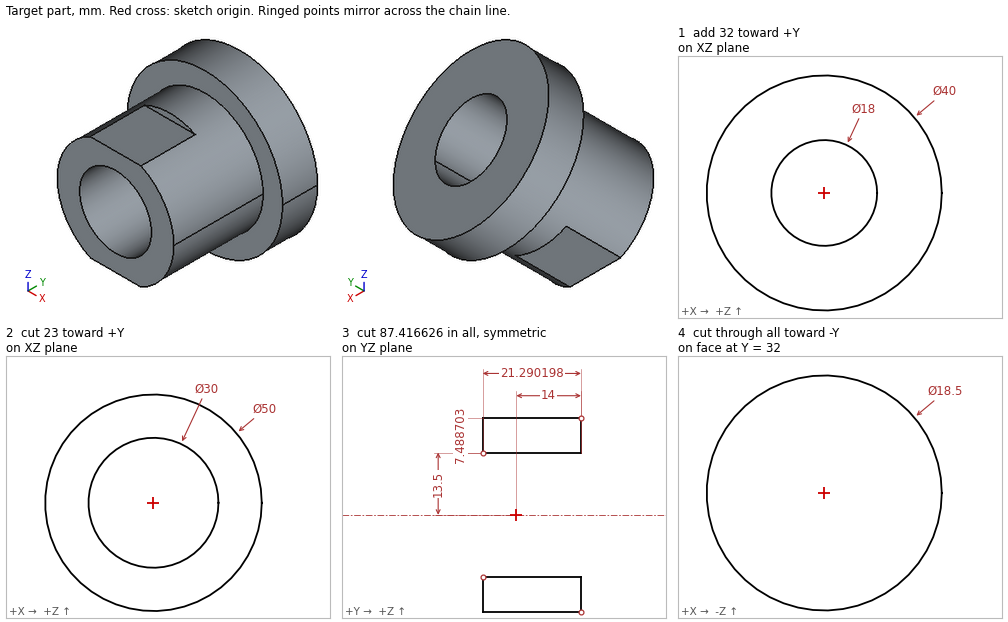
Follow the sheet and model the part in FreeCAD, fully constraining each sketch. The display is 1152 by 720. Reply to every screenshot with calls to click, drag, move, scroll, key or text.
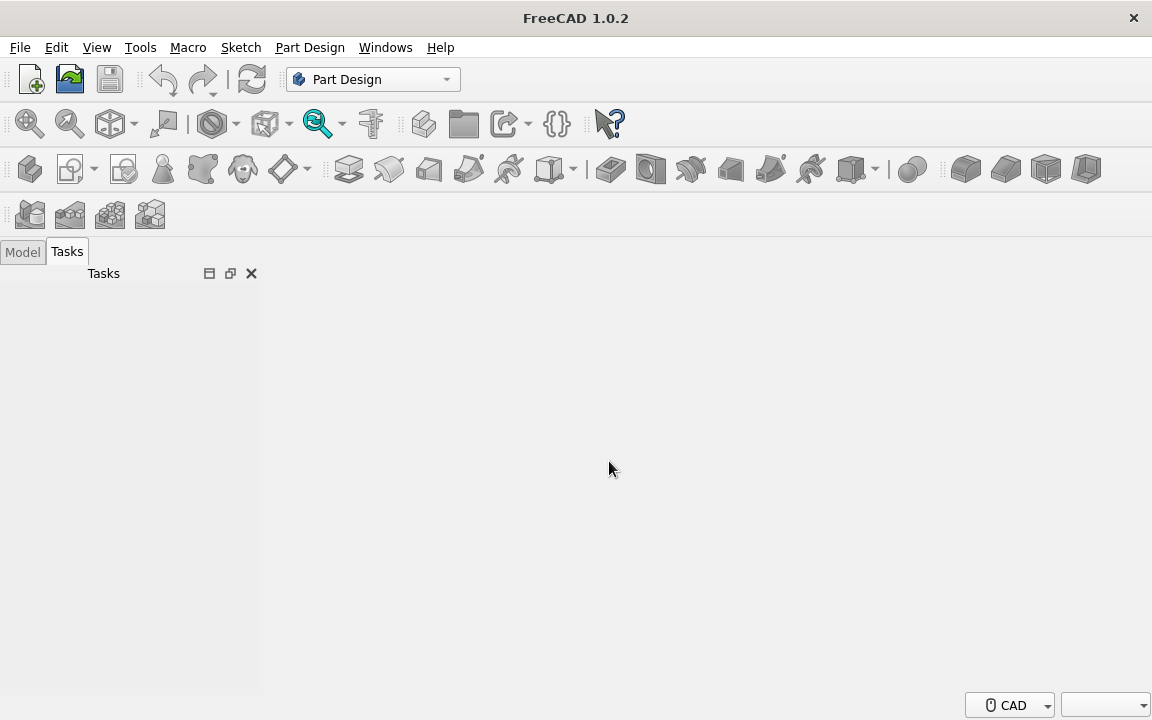
key(ctrl+n)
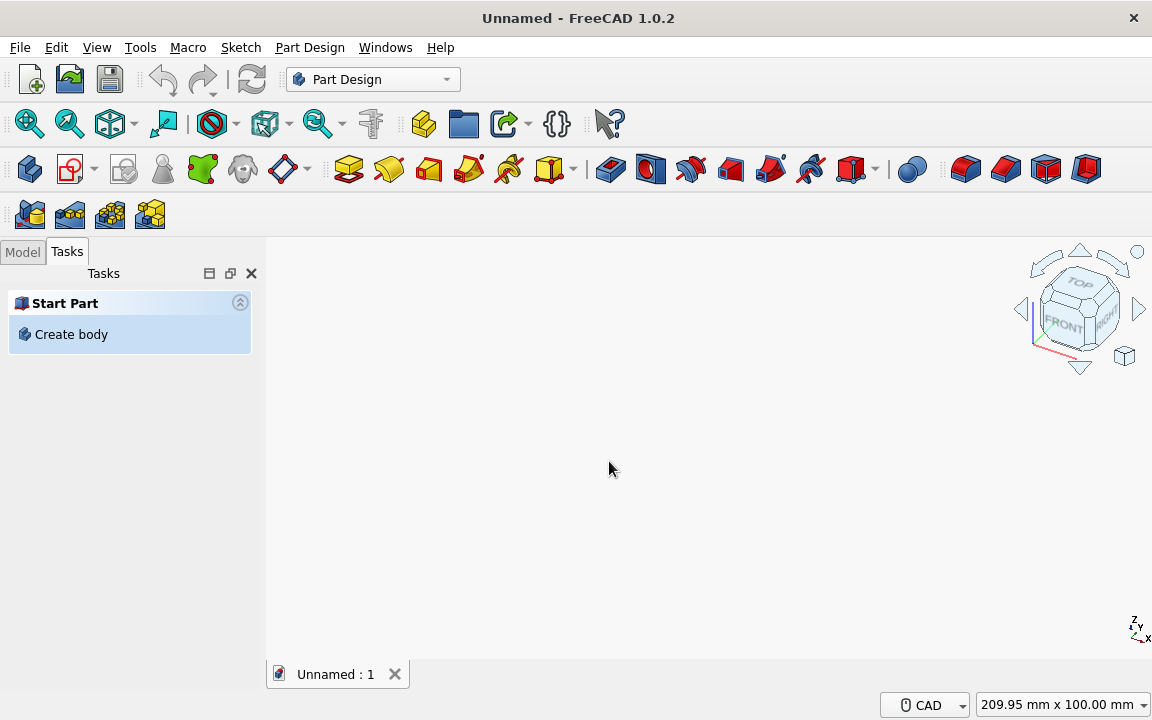
click(70, 170)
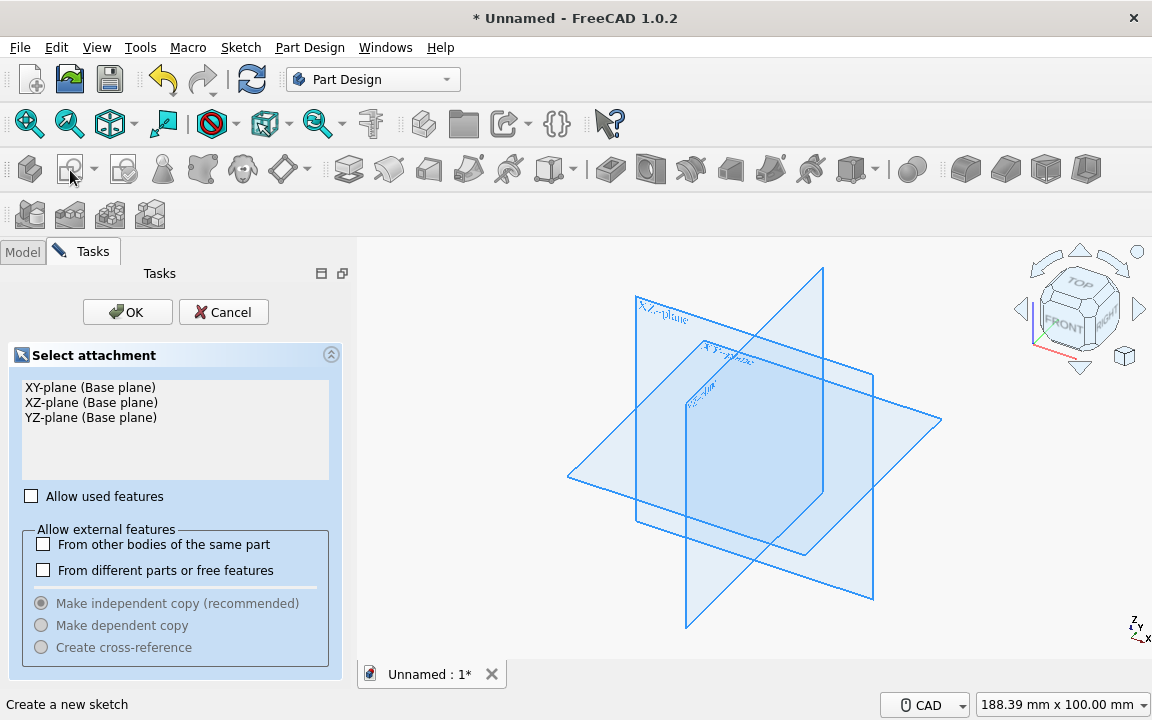
click(82, 402)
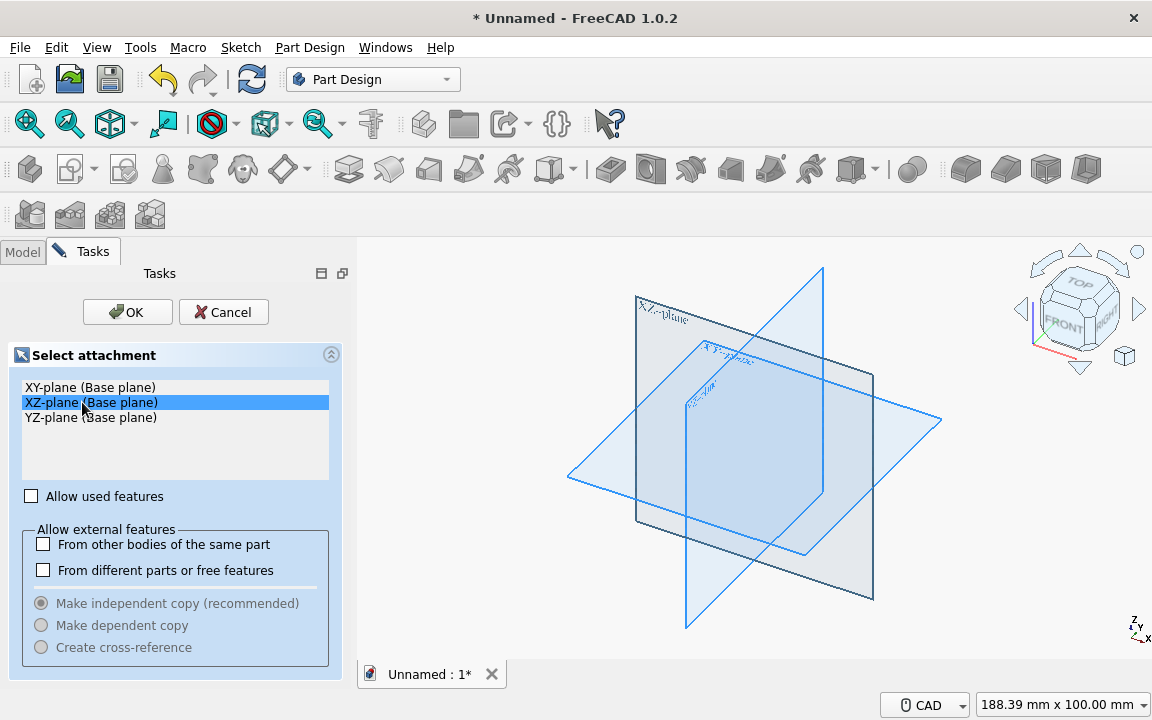
click(128, 312)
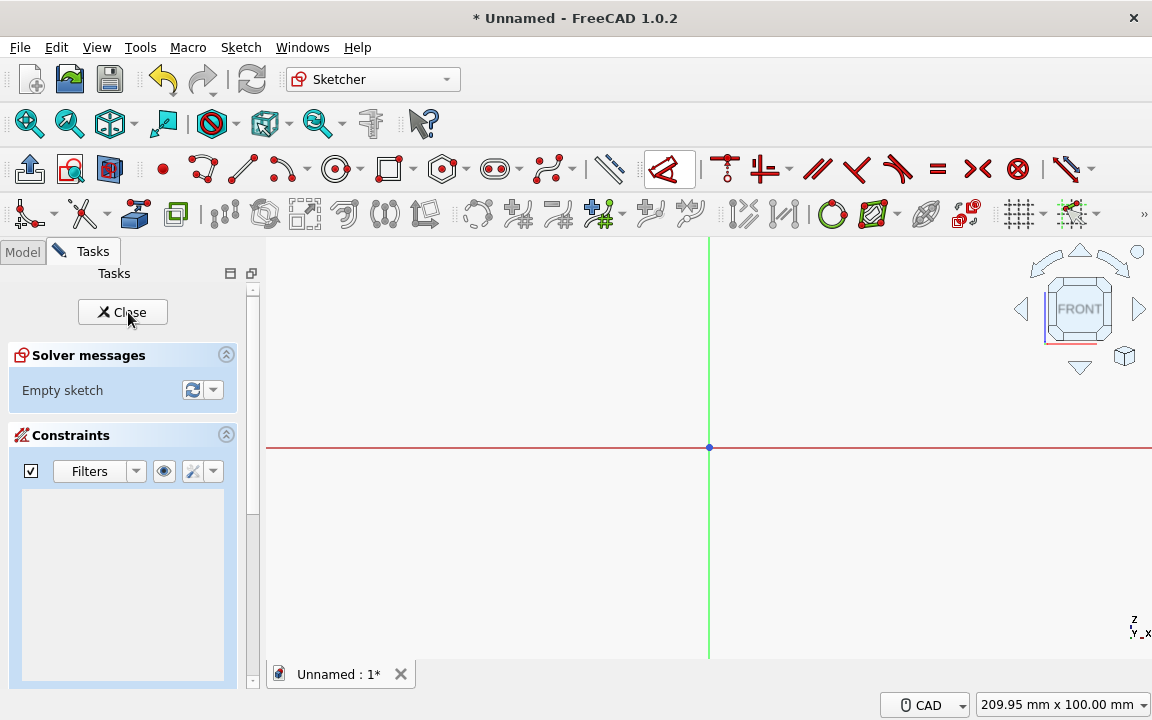
scroll(848, 448, up, 2)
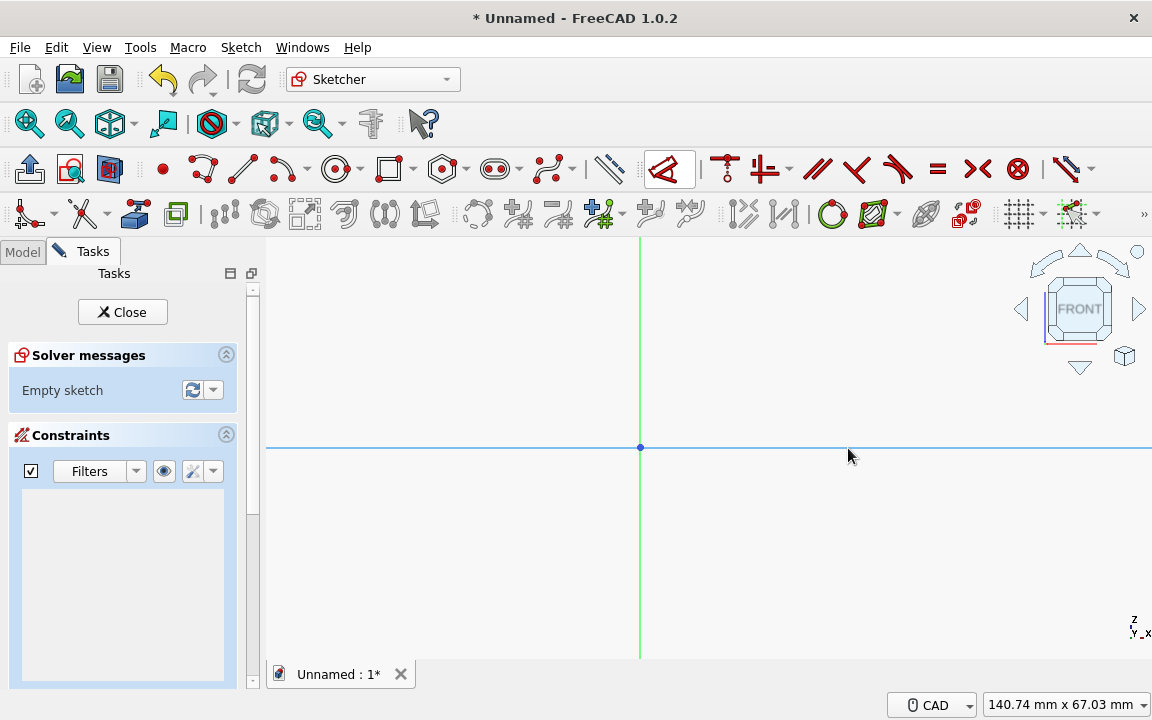
click(336, 170)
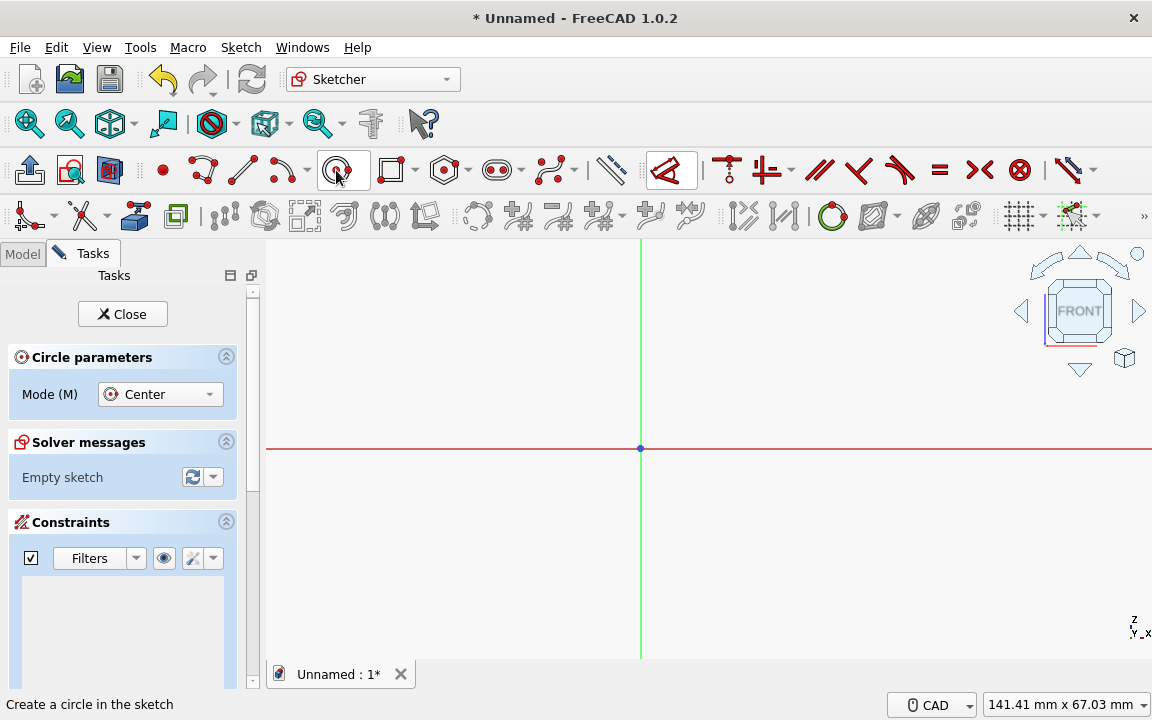
click(641, 449)
click(729, 360)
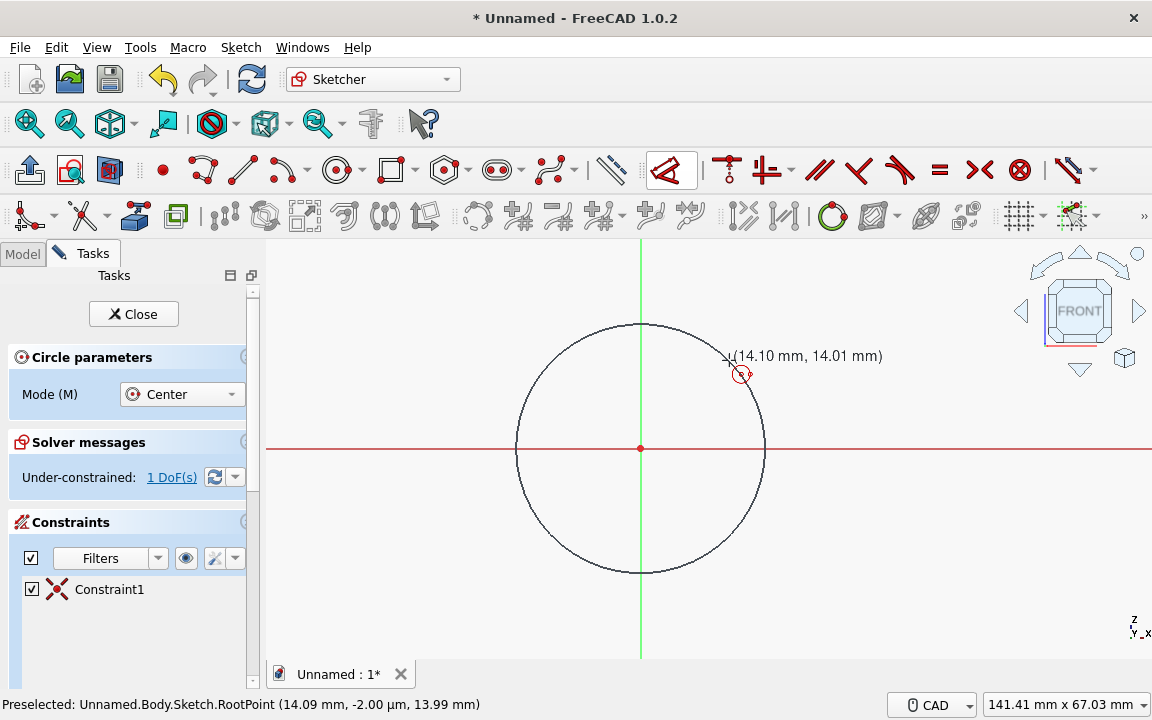
click(641, 449)
click(681, 409)
key(Escape)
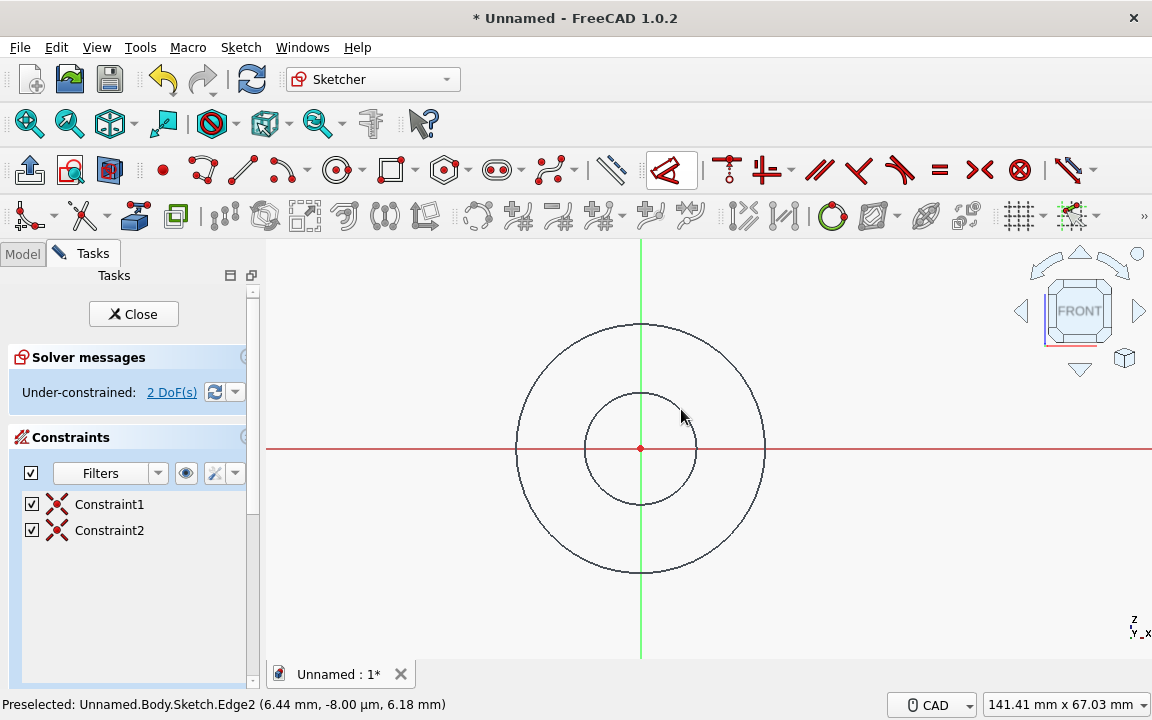
click(728, 360)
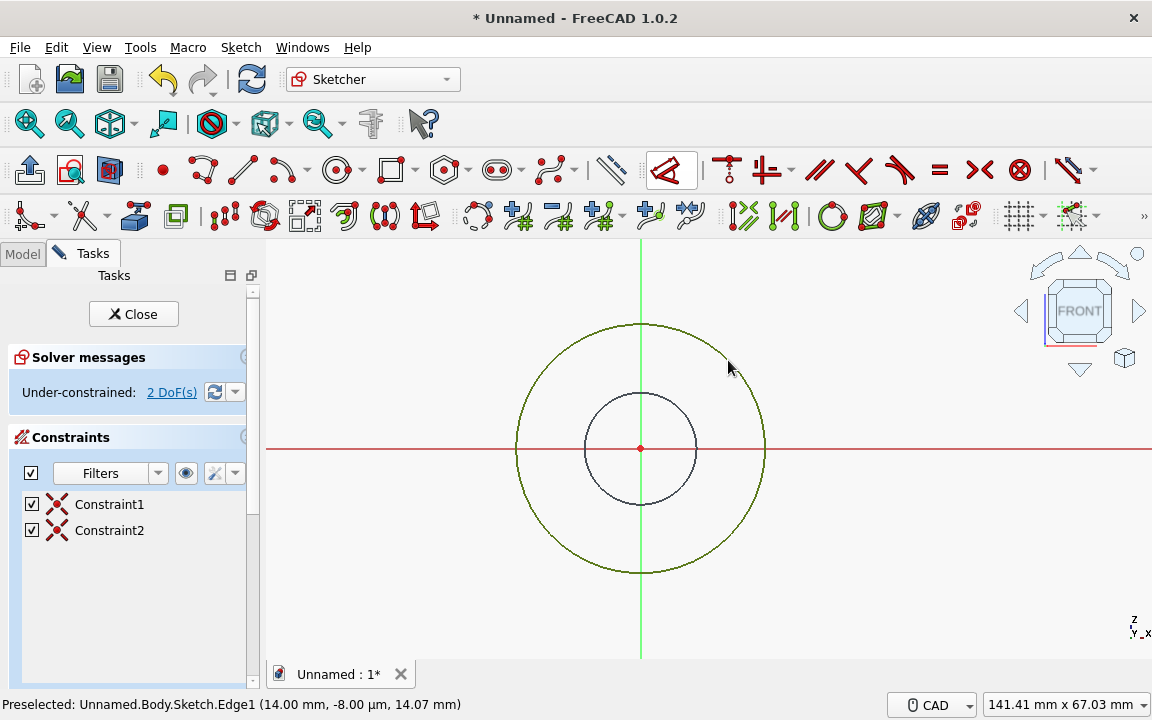
click(692, 170)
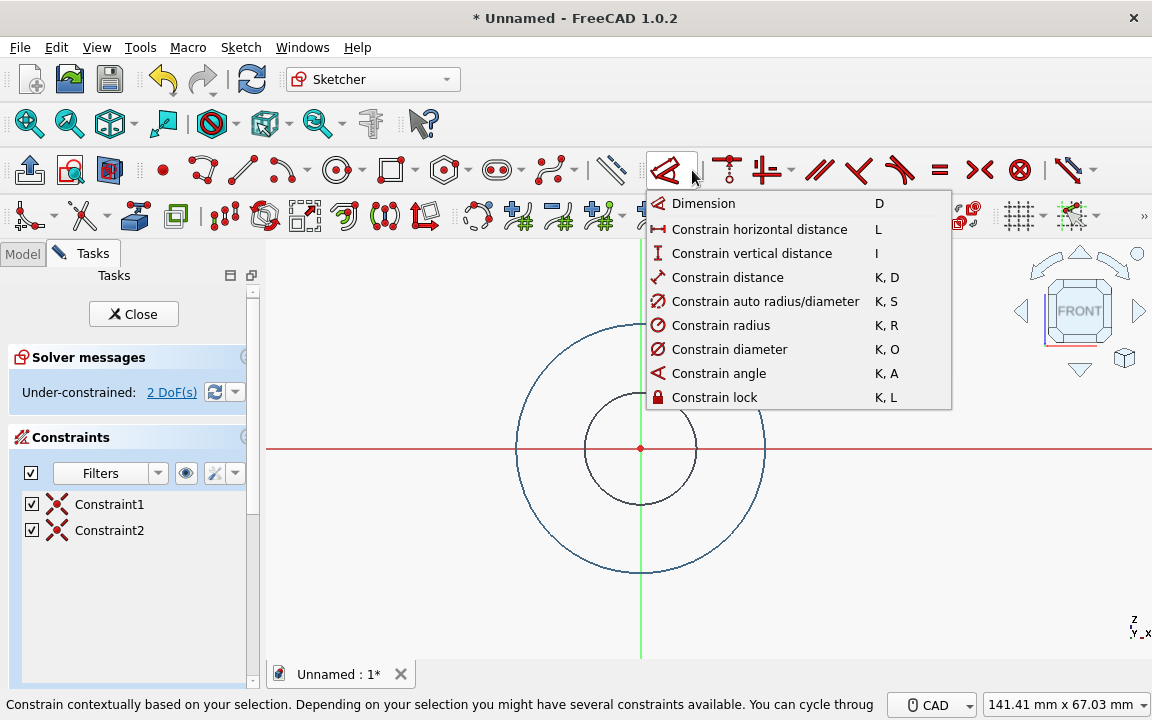
click(799, 349)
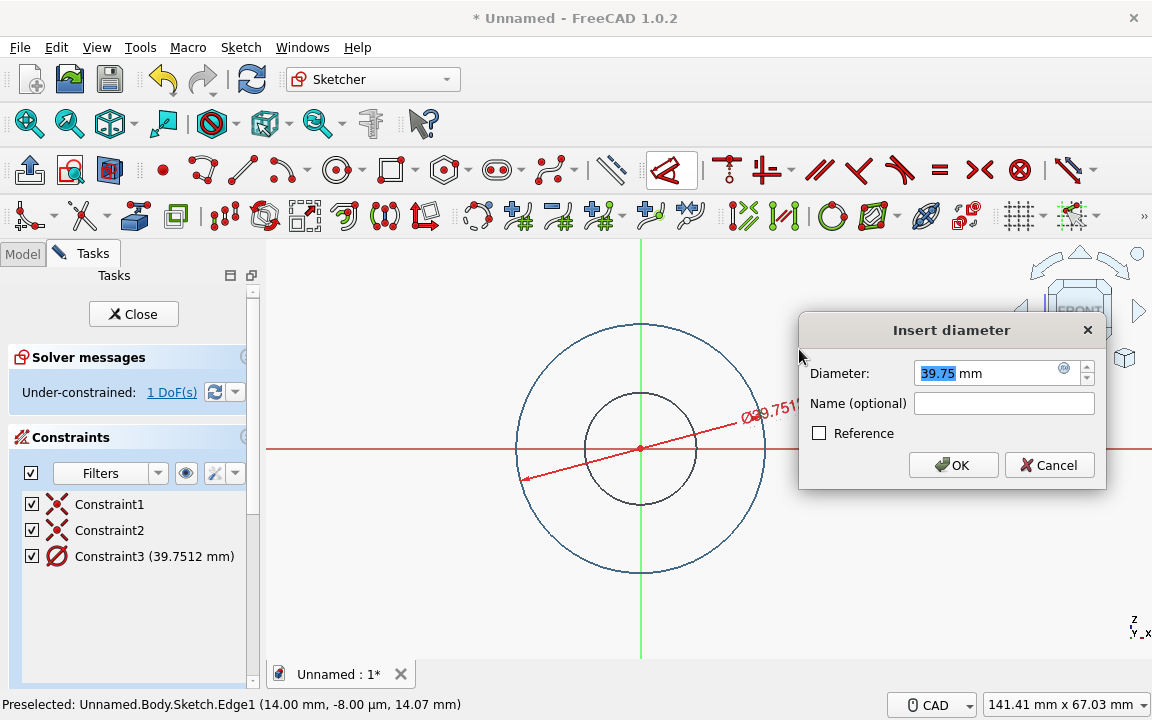
text(40)
key(Return)